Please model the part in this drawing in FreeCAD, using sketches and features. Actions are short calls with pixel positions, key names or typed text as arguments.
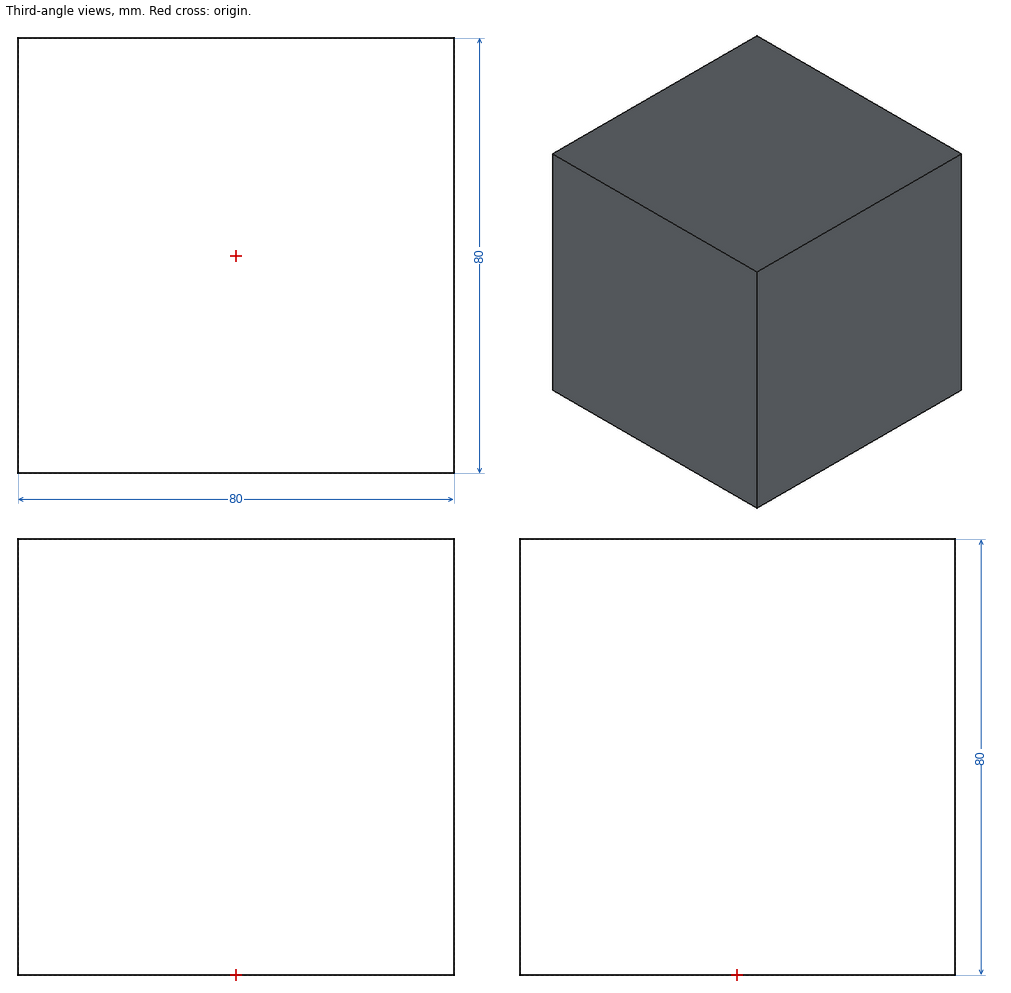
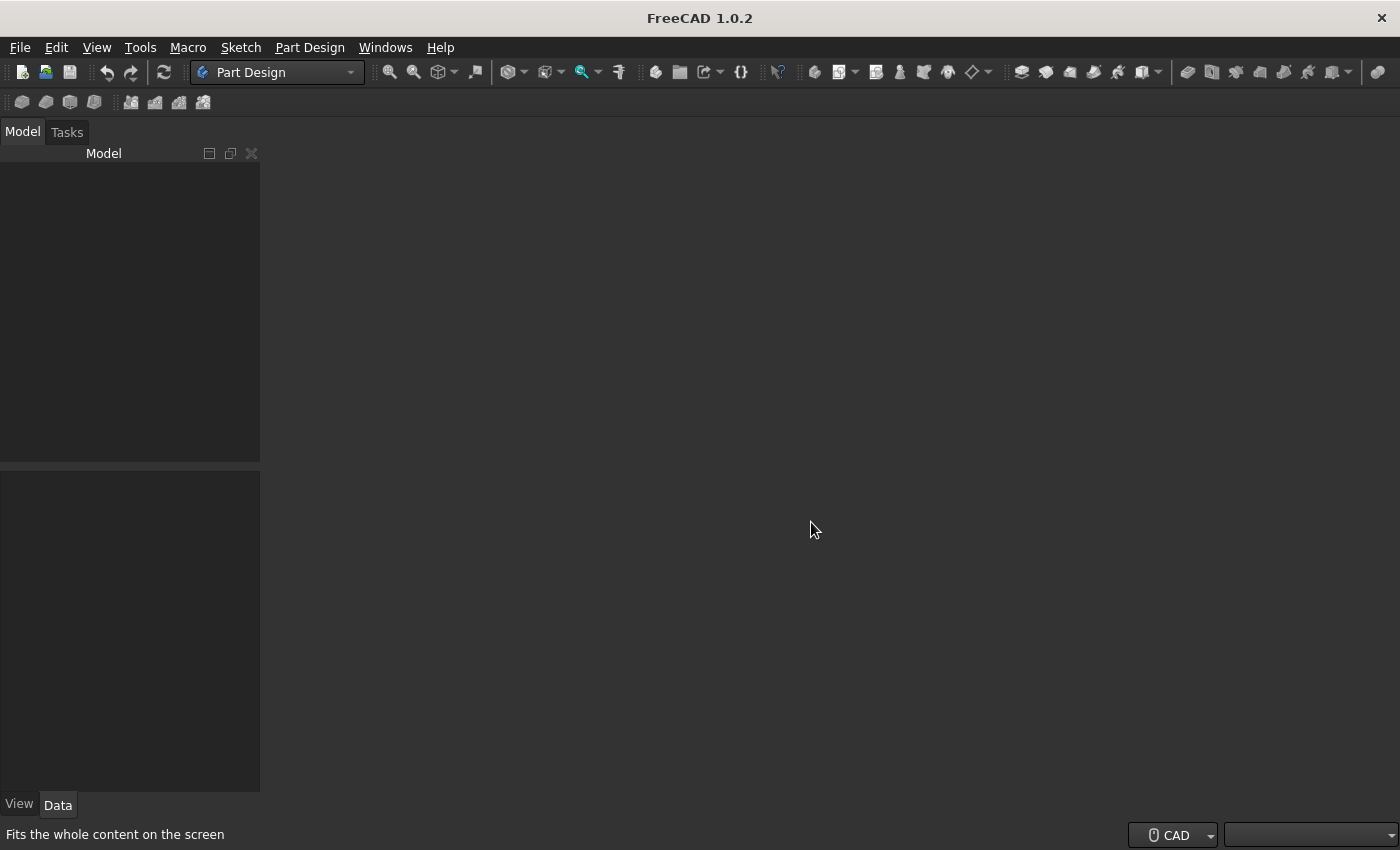
key(ctrl+n)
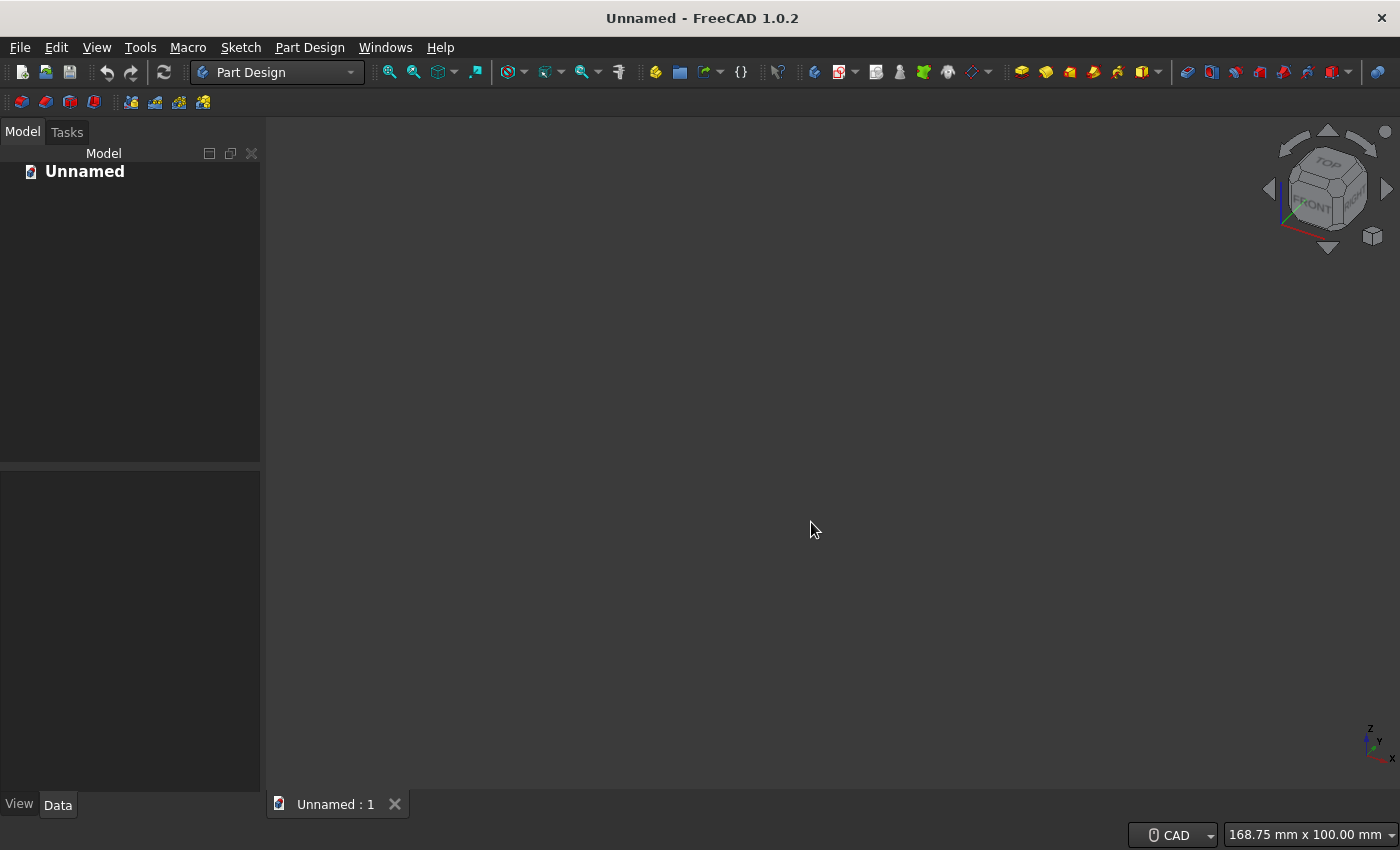
click(840, 72)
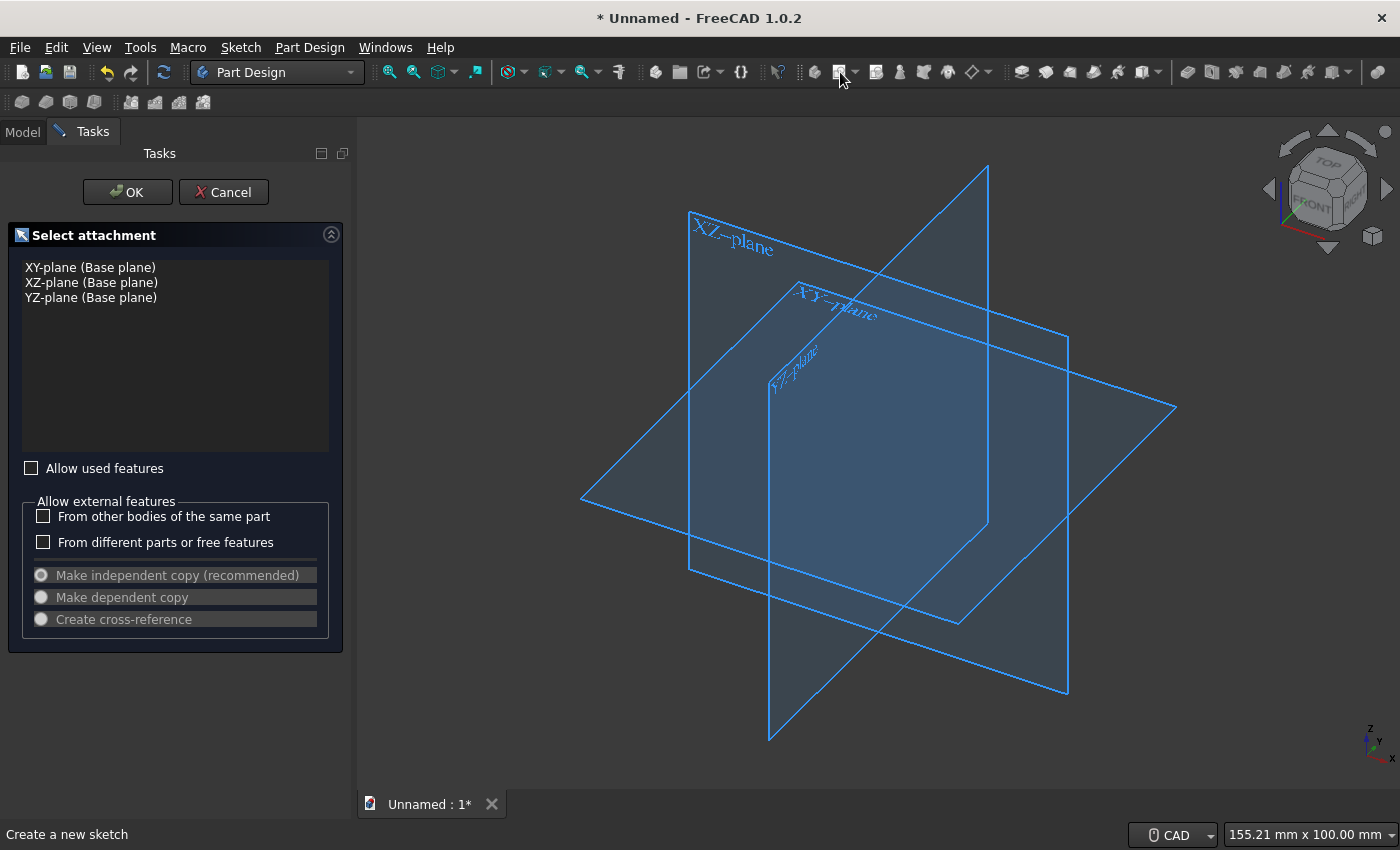
click(82, 268)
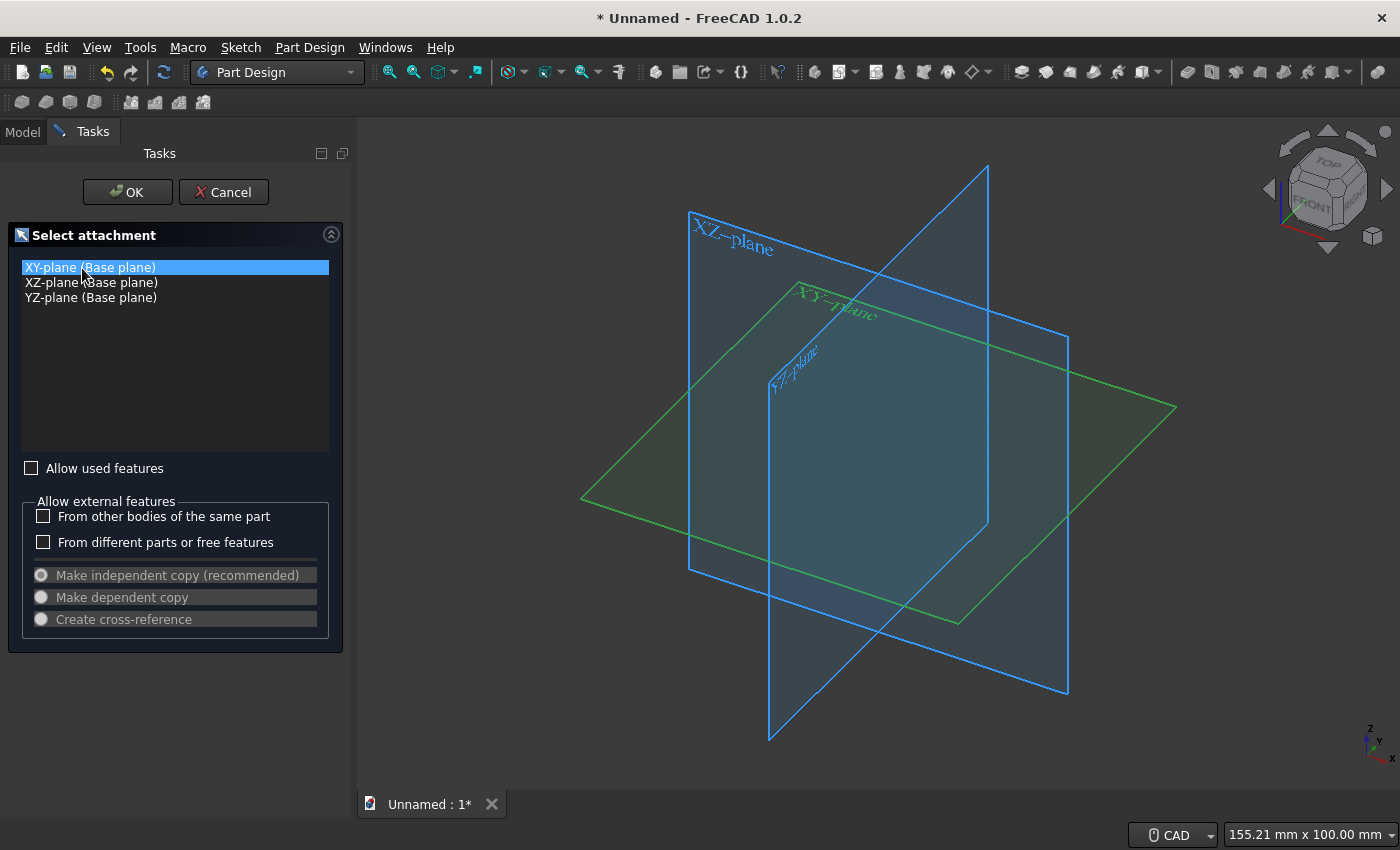
click(128, 192)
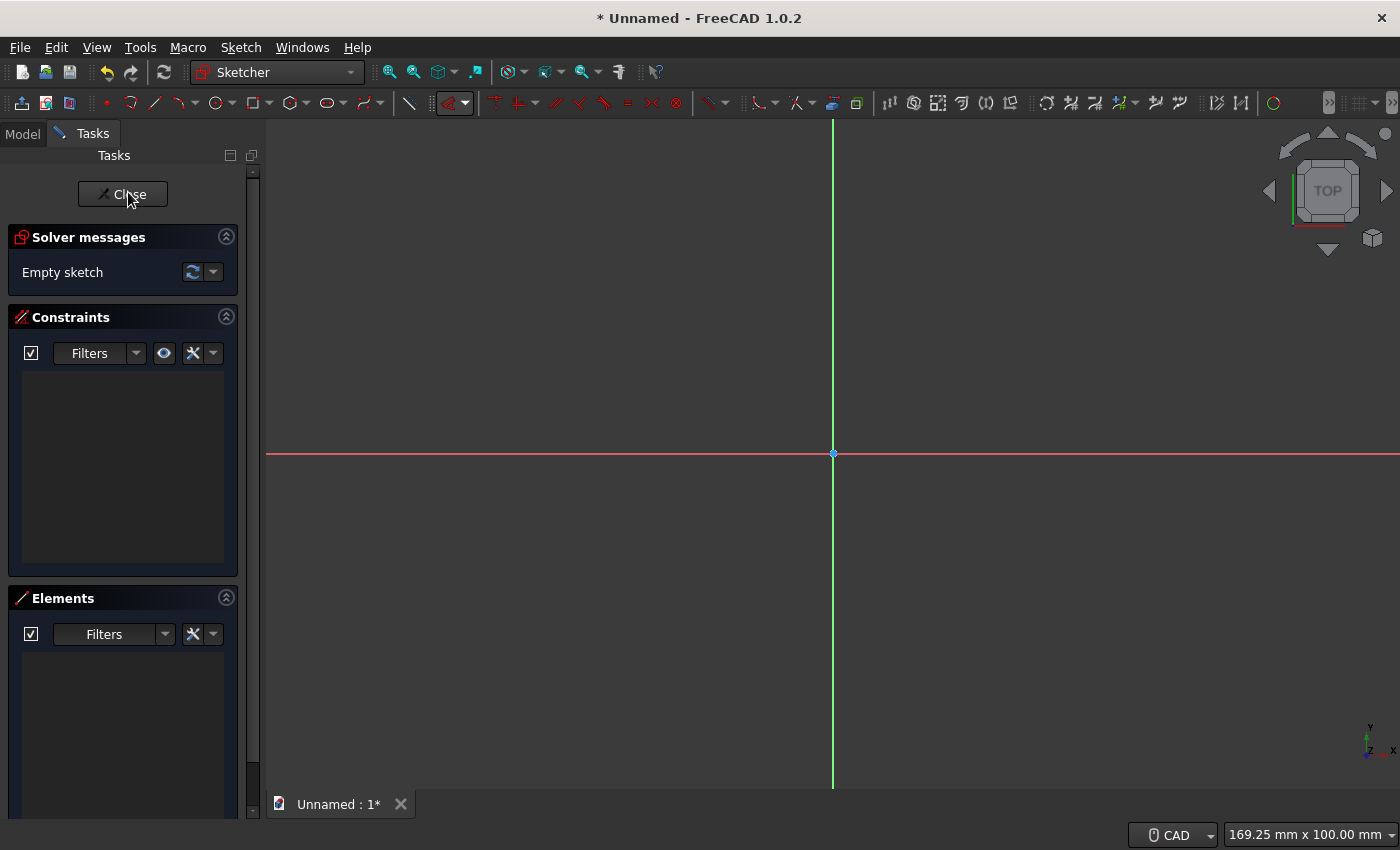
key(g)
key(v)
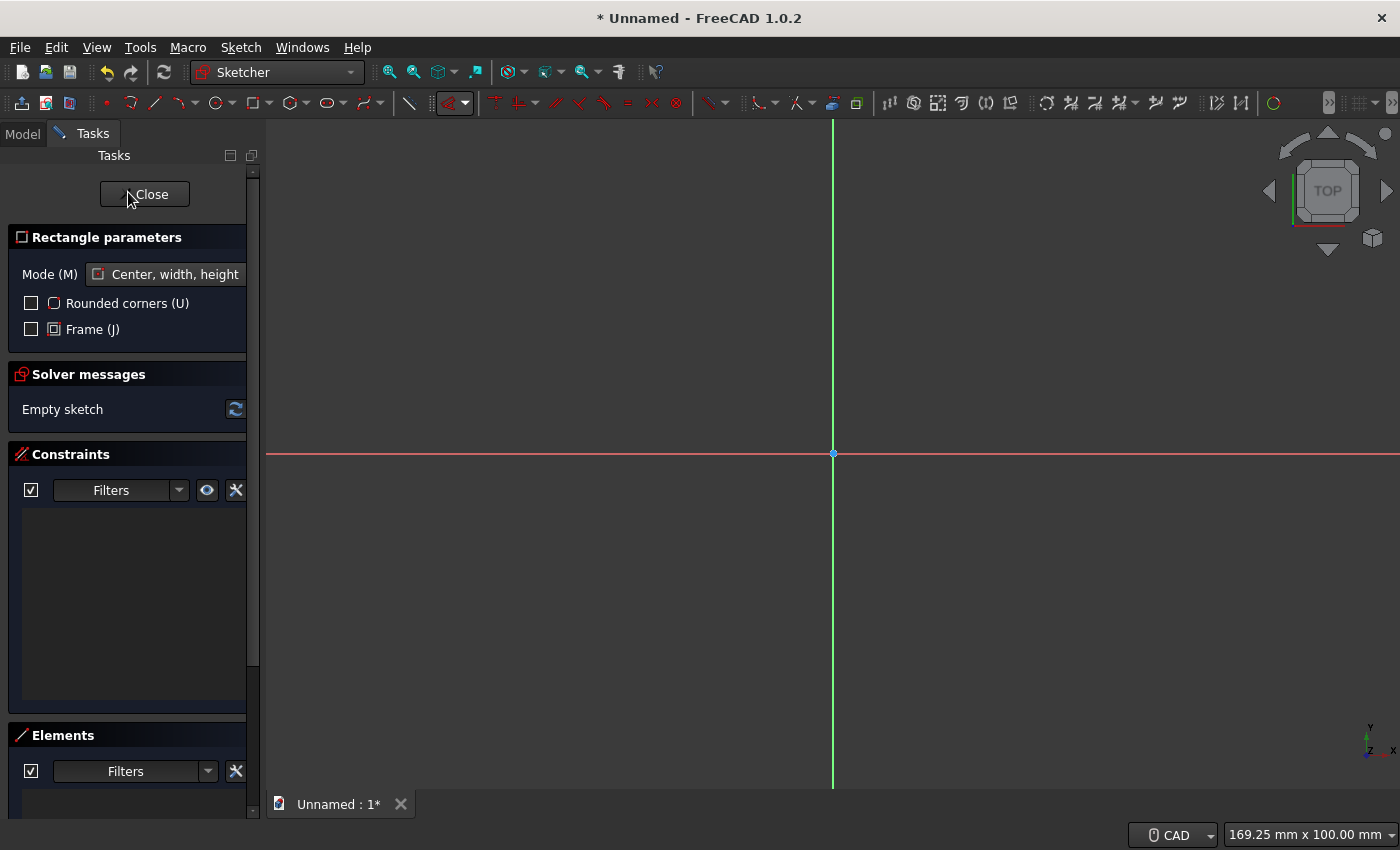
click(833, 454)
move(1101, 186)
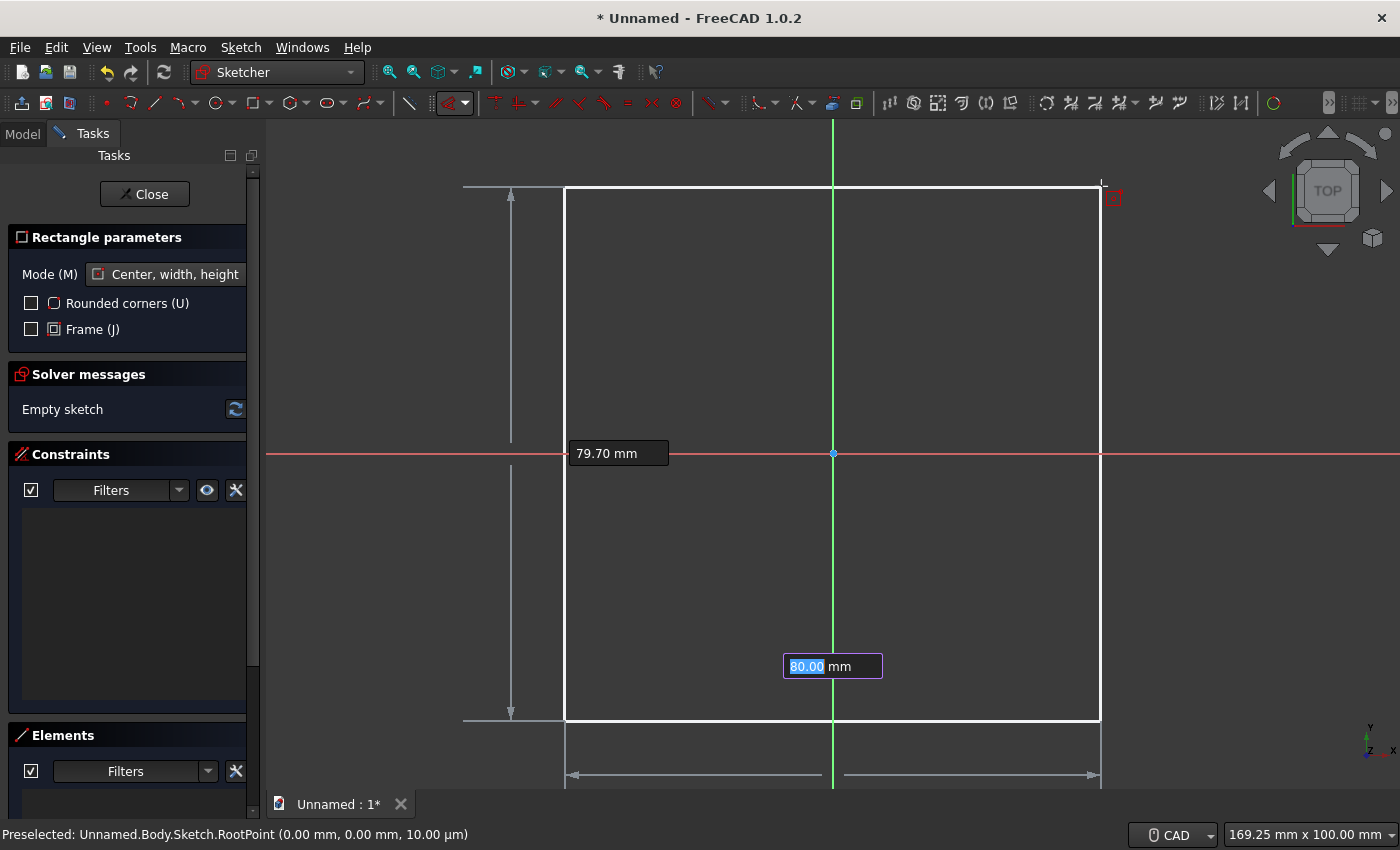
text(80)
key(Tab)
text(80)
key(Return)
key(Escape)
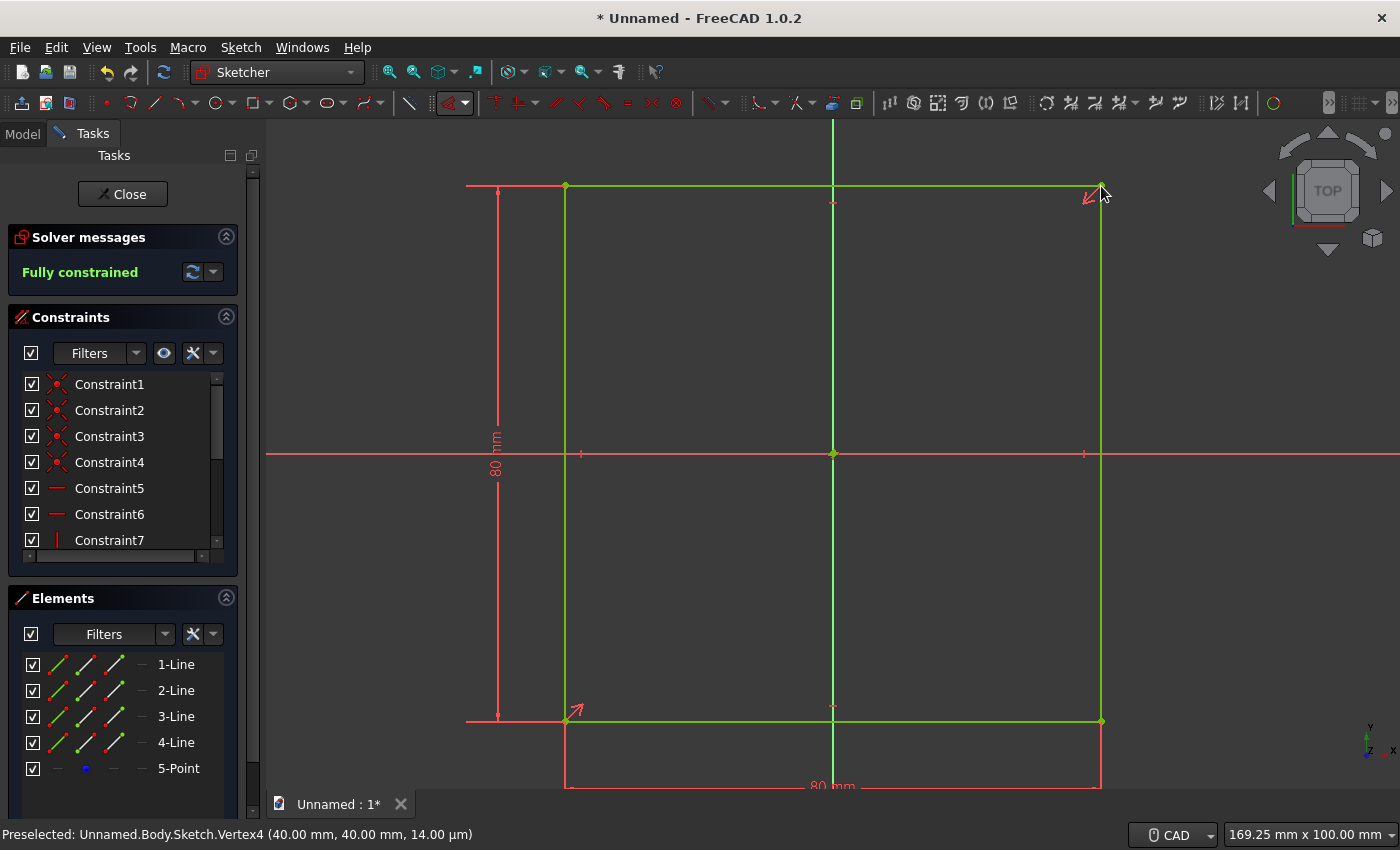
click(123, 194)